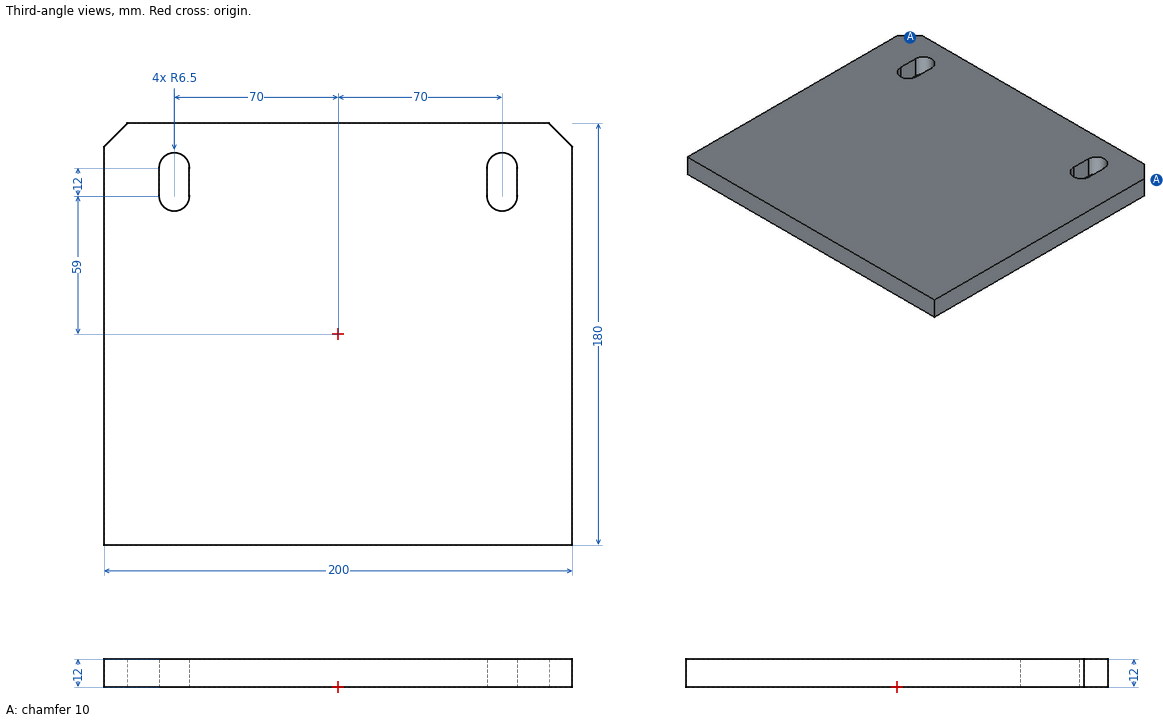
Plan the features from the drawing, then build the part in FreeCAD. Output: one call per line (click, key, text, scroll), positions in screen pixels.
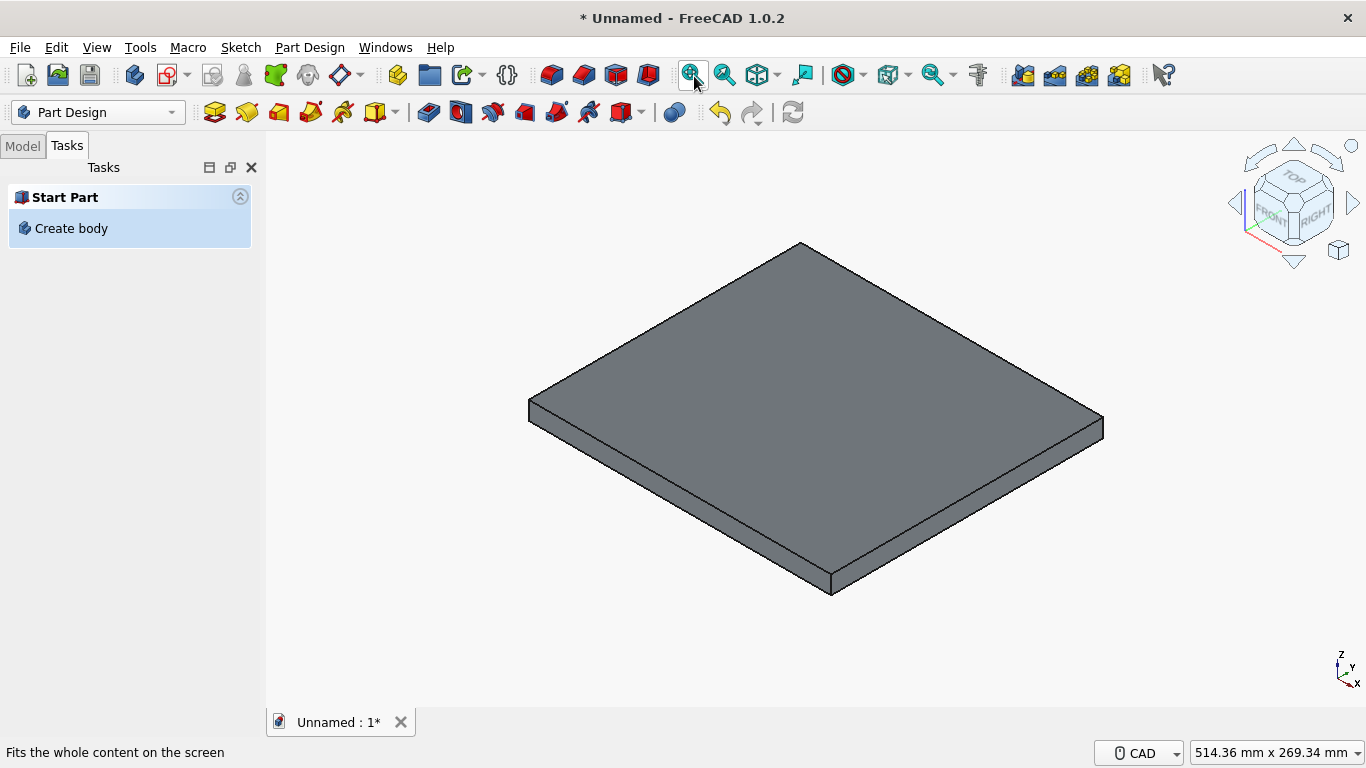
key(2)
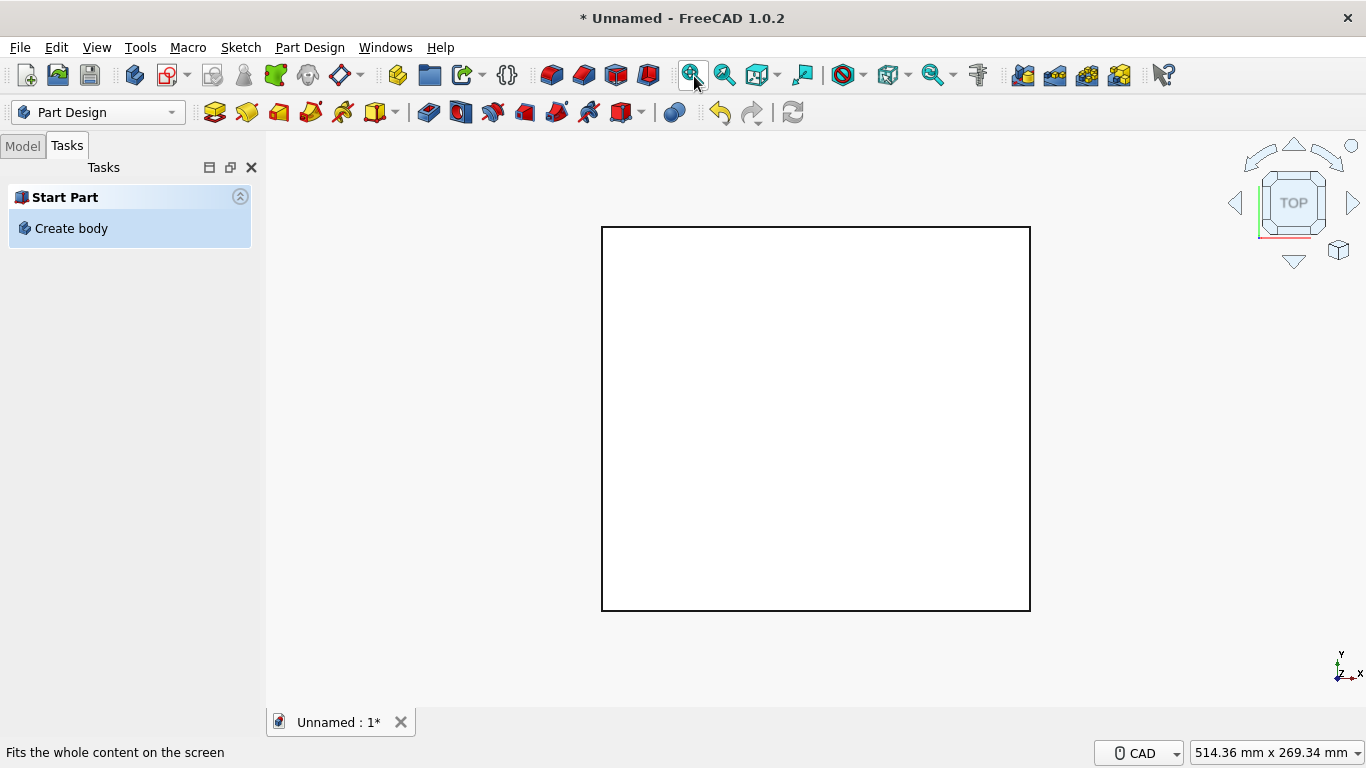
key(1)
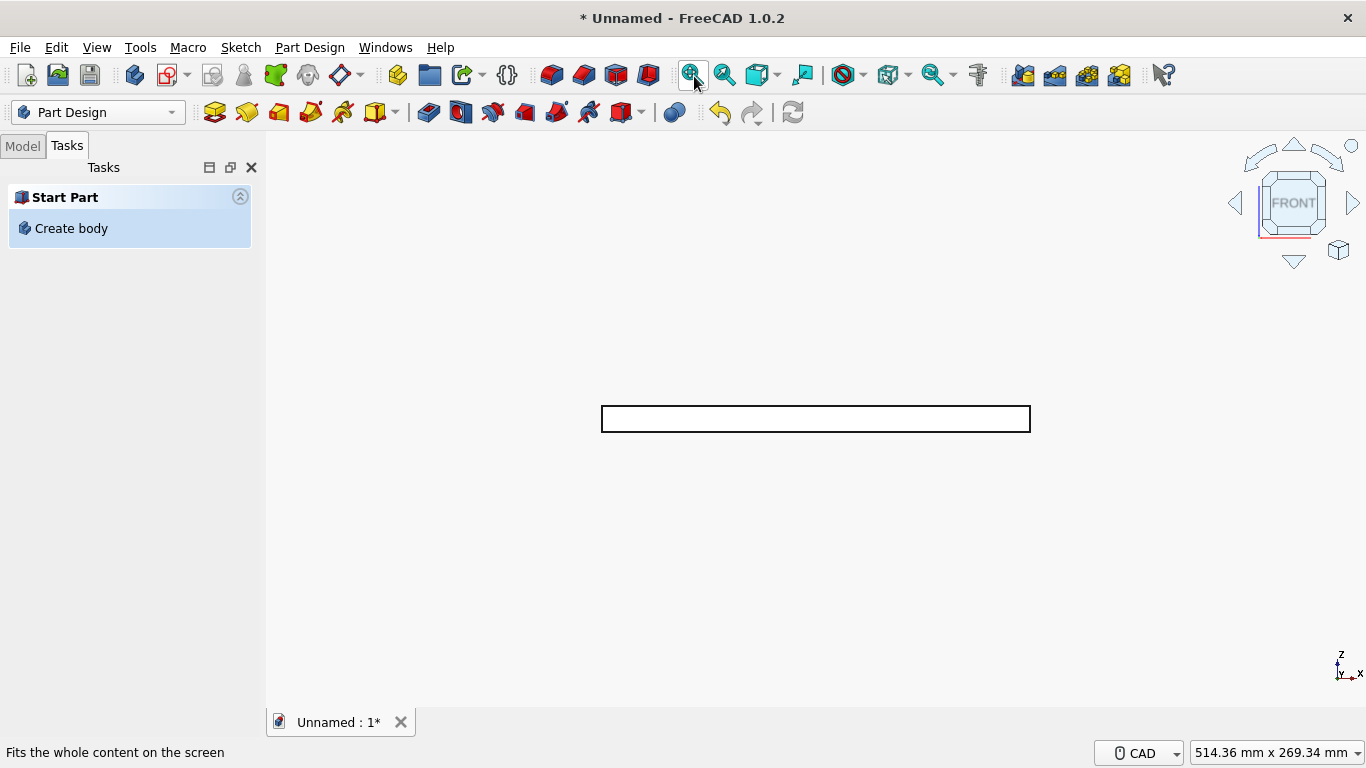
click(694, 76)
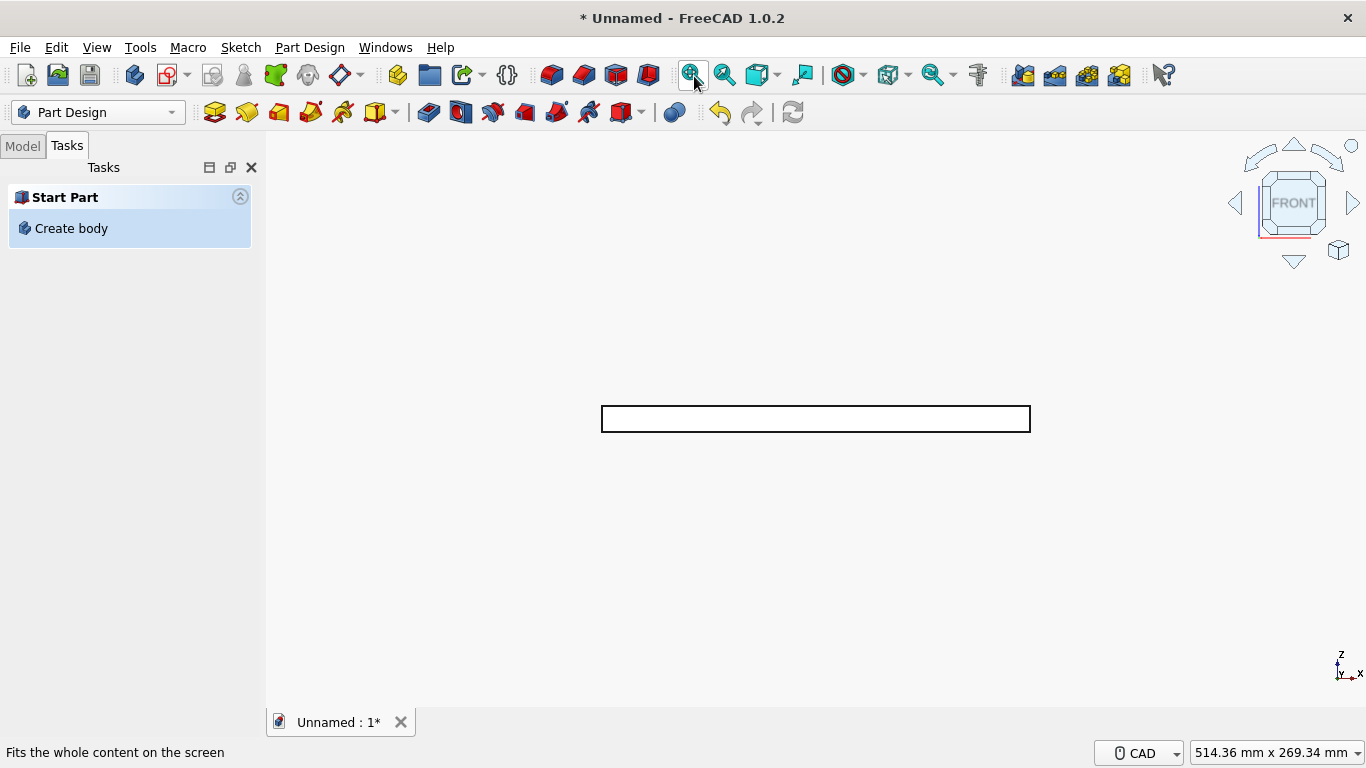
key(3)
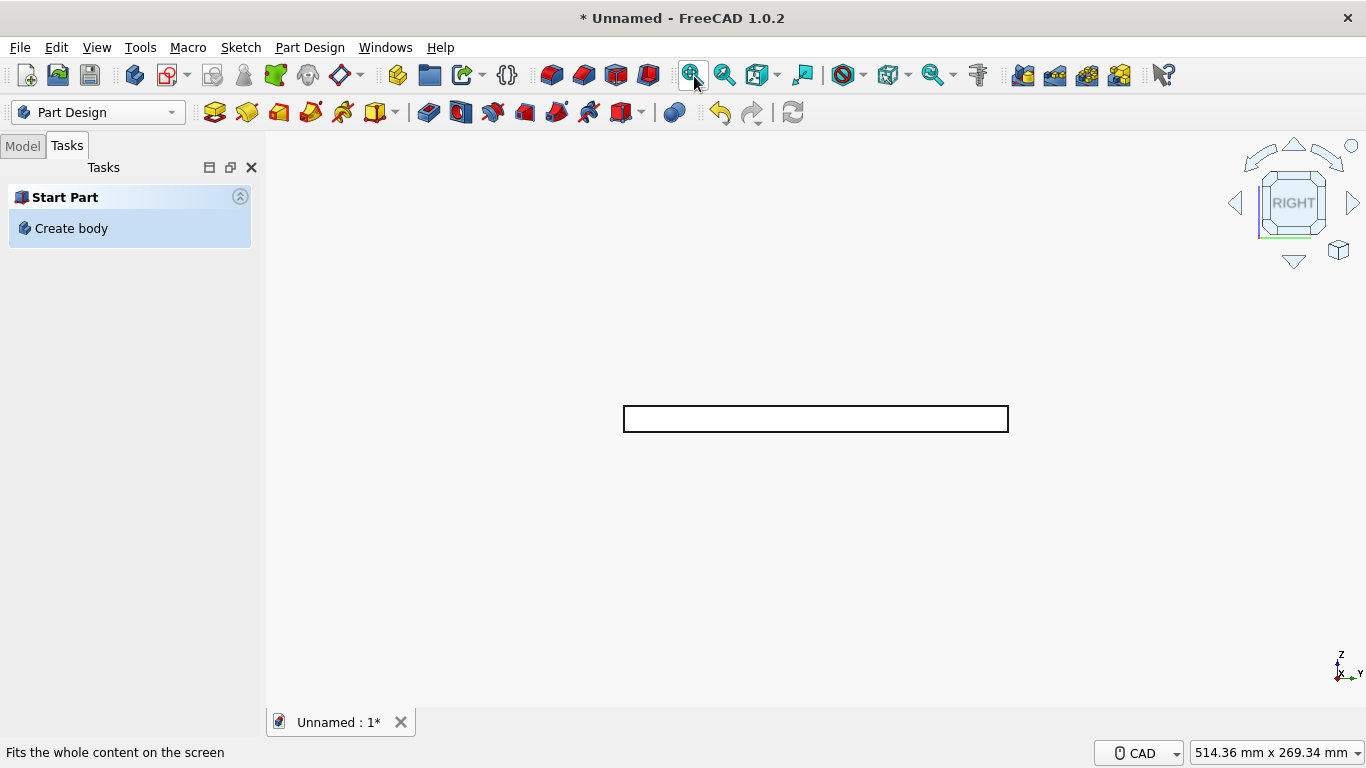
key(v)
key(f)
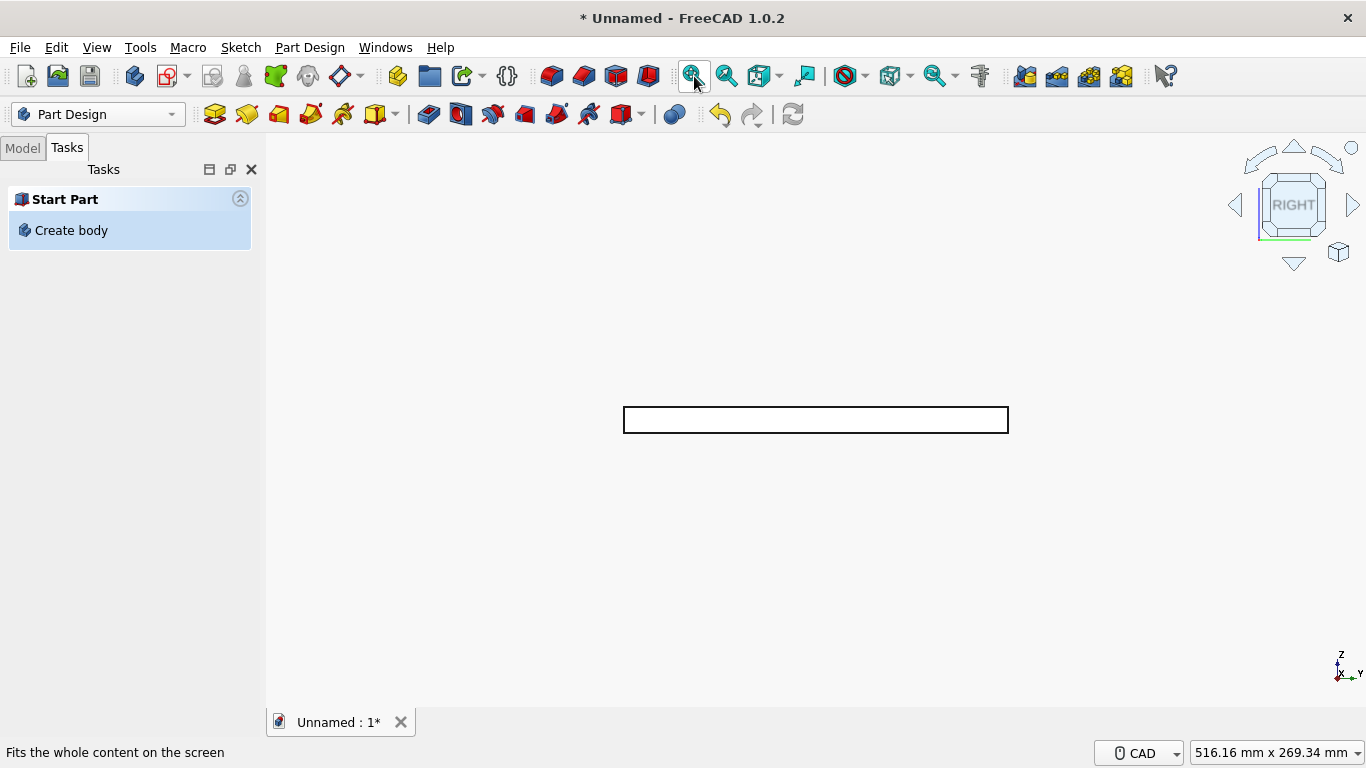
click(1008, 419)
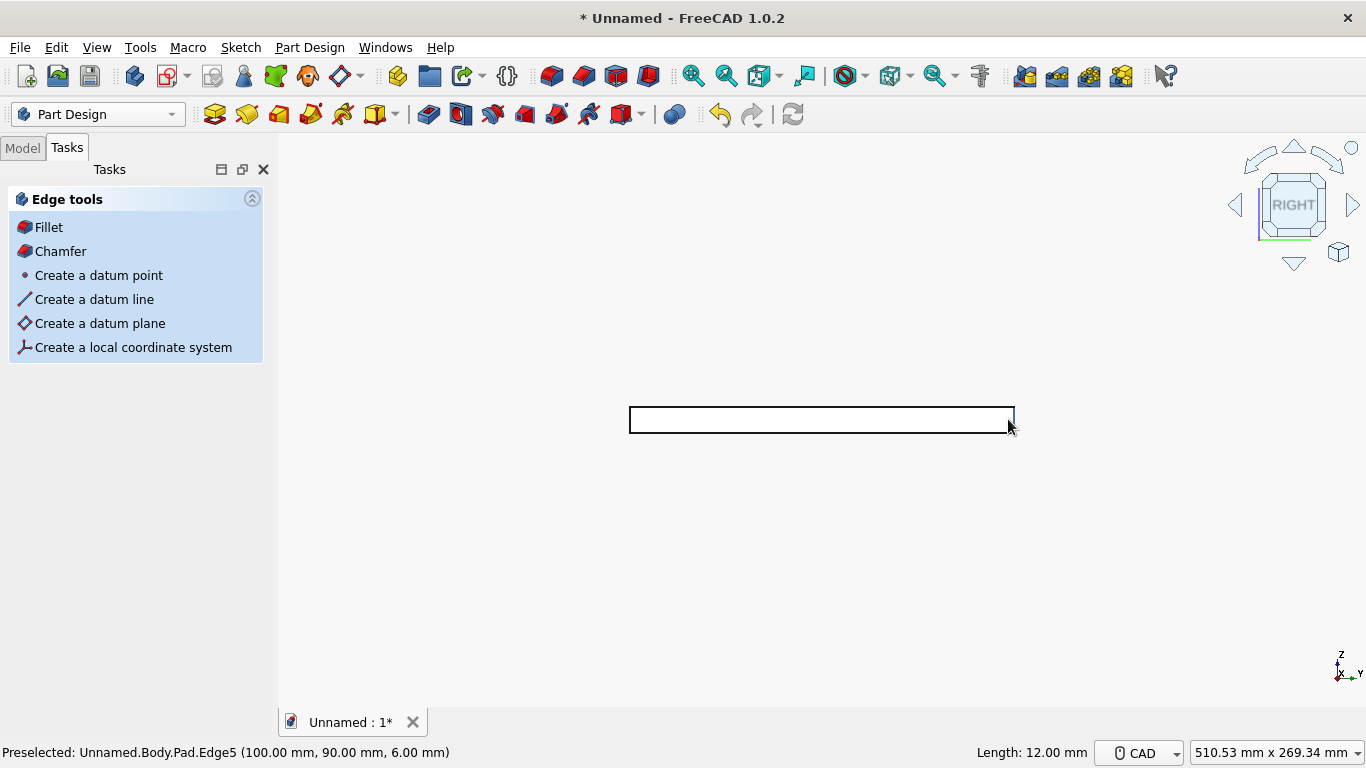
key(5)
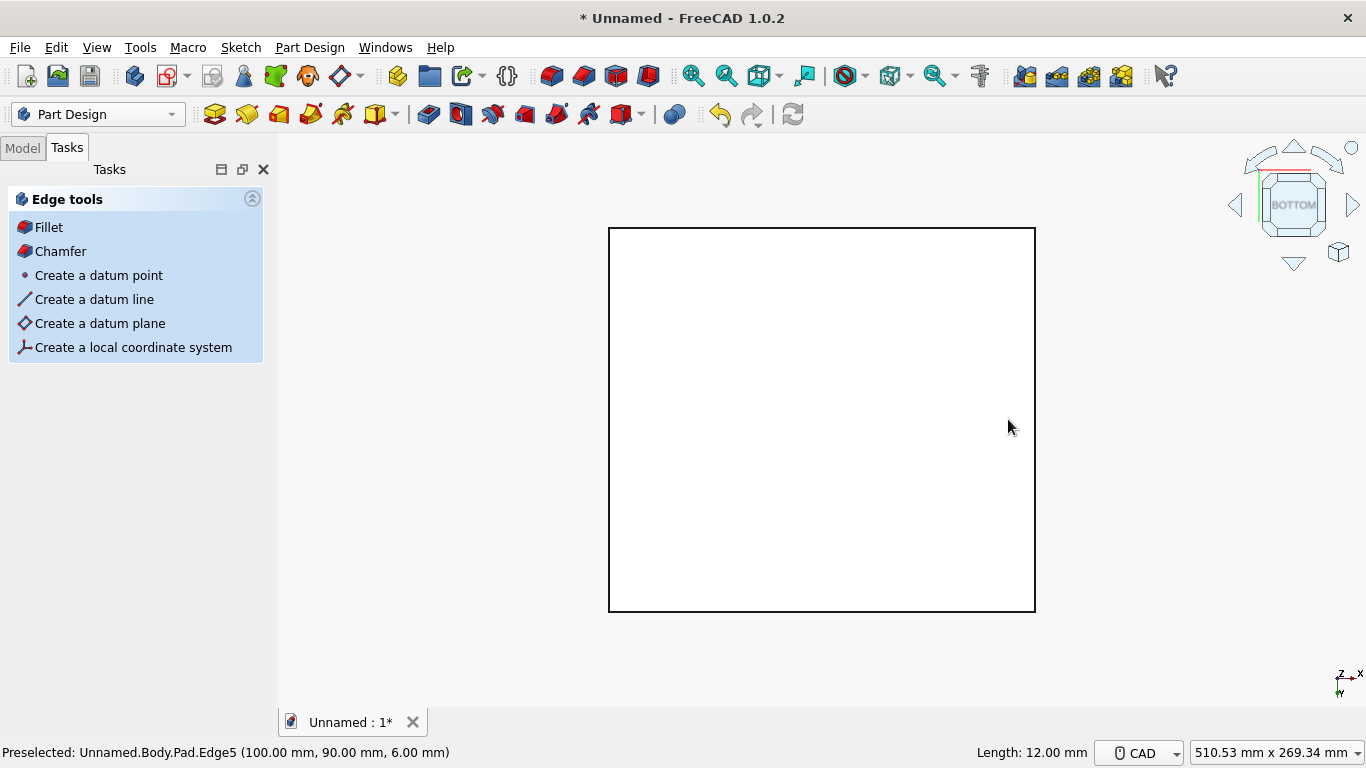
key(4)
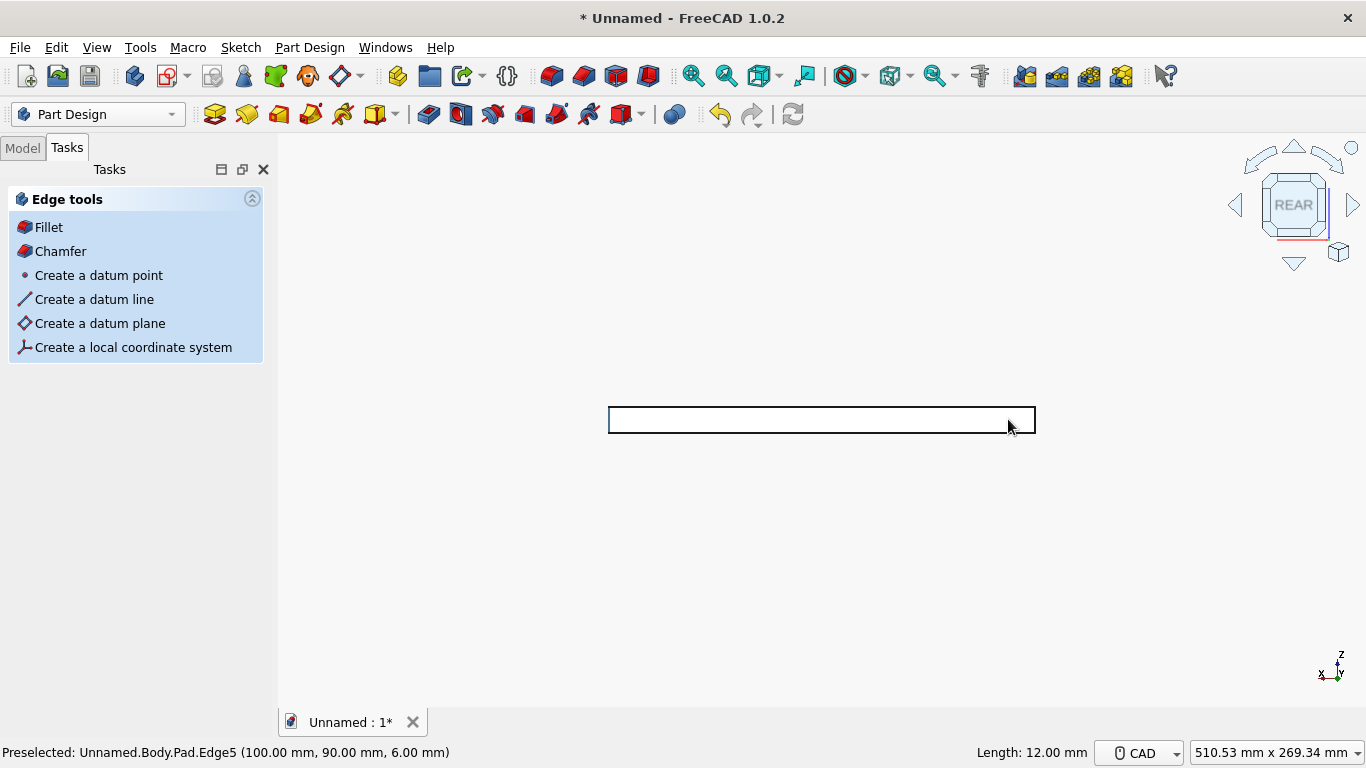
click(694, 76)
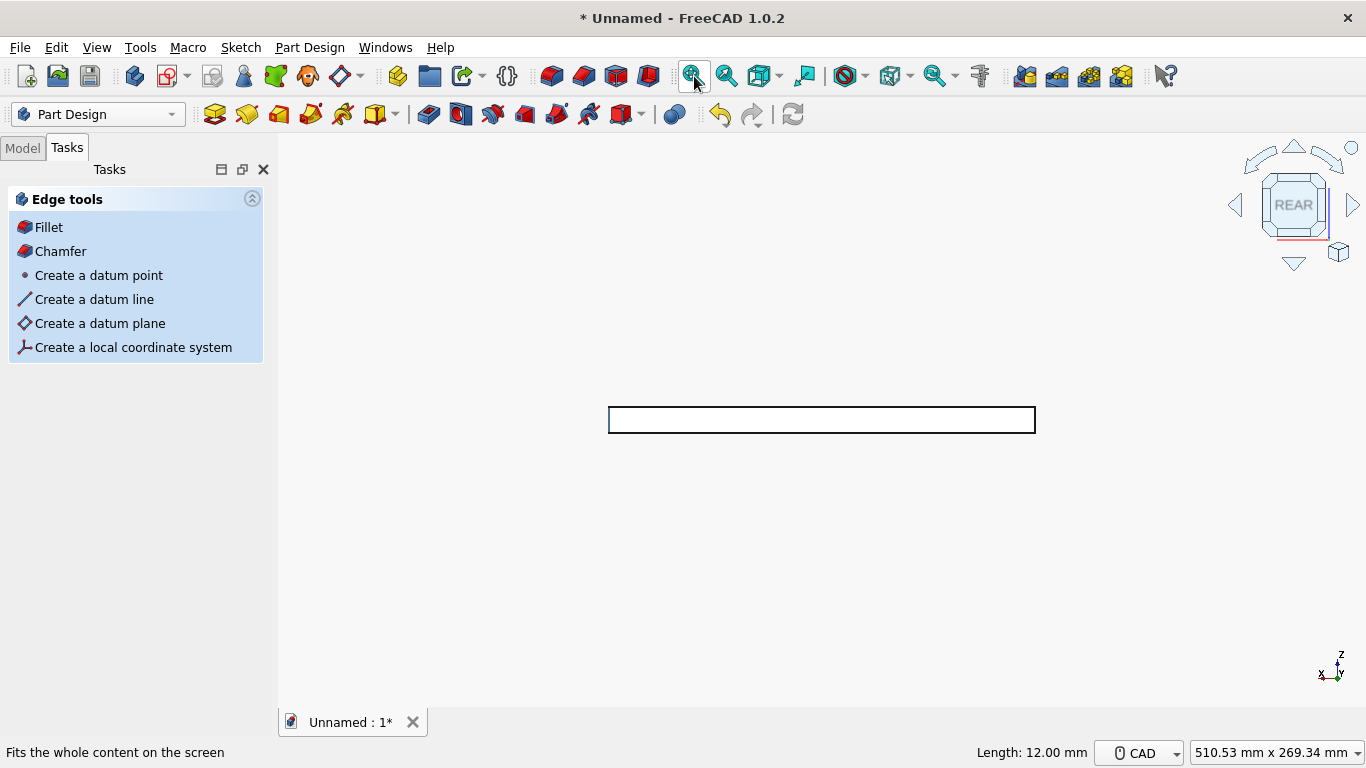
click(1035, 419, ctrl)